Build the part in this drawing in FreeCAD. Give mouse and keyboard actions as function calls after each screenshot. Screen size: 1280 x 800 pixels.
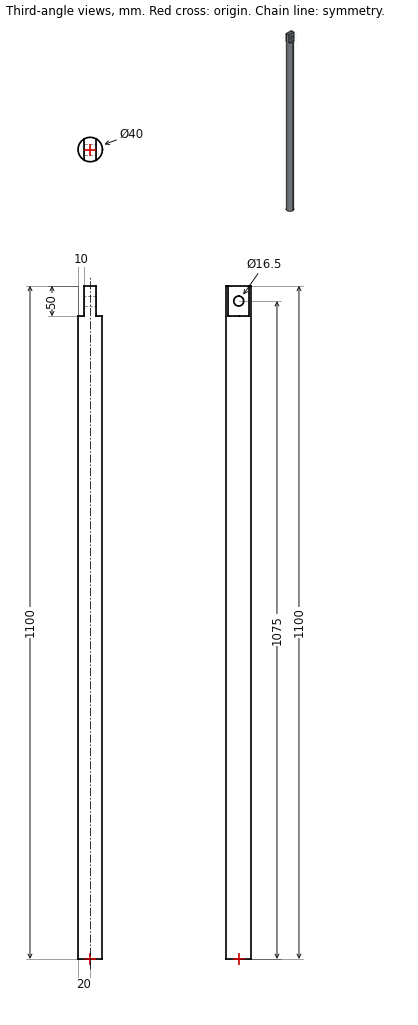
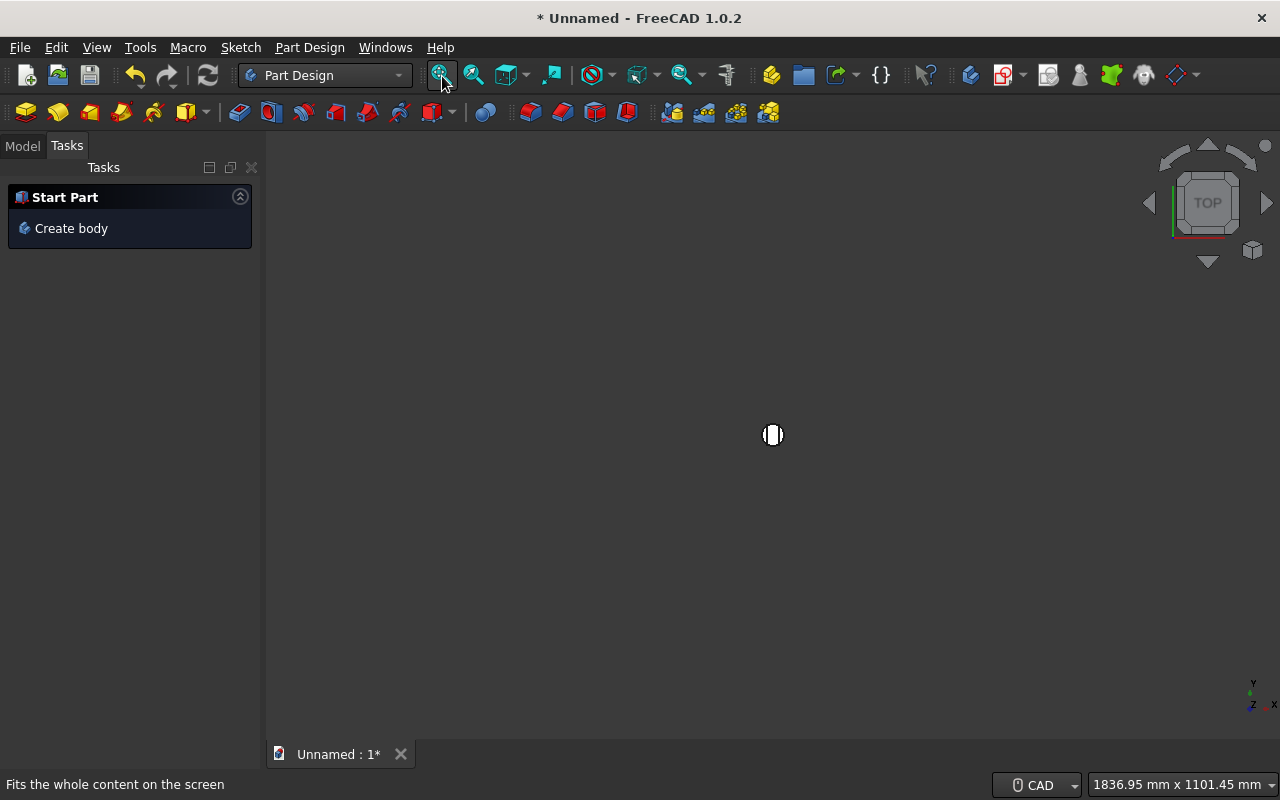
click(442, 76)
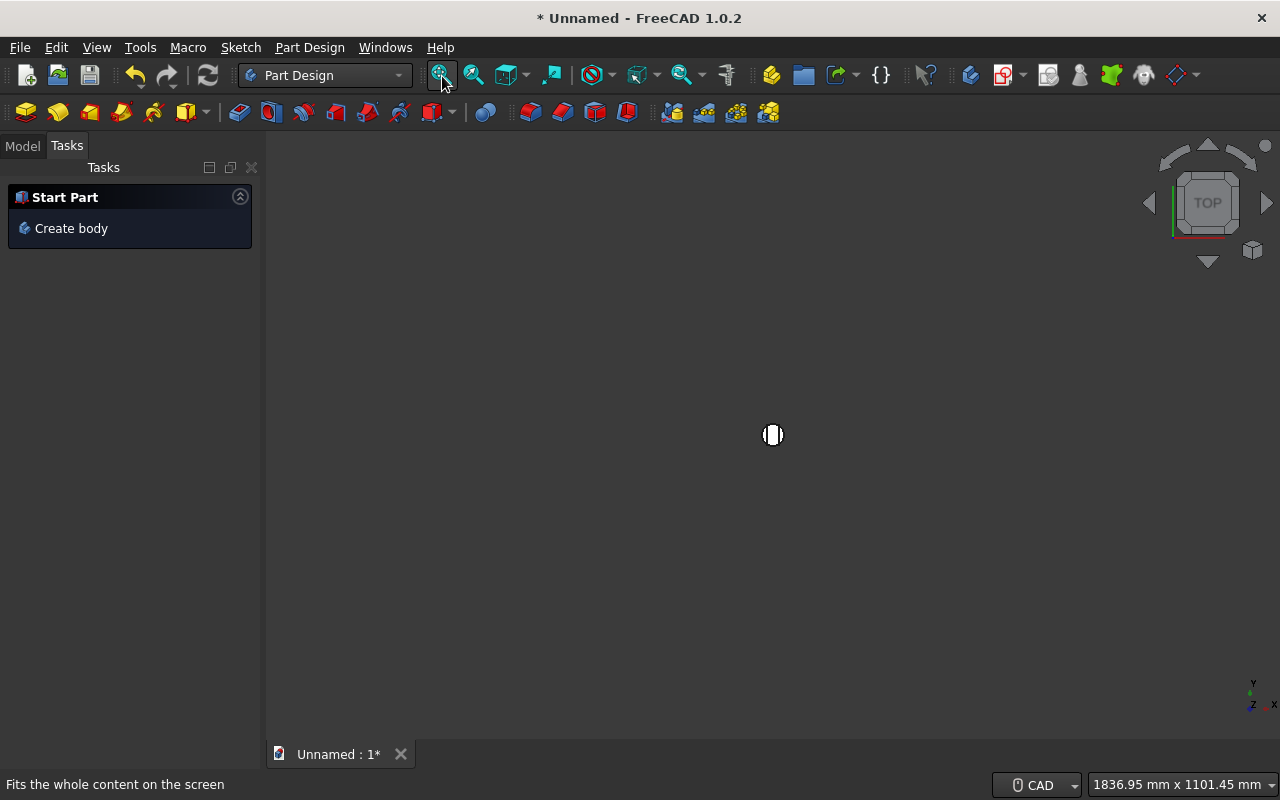
key(1)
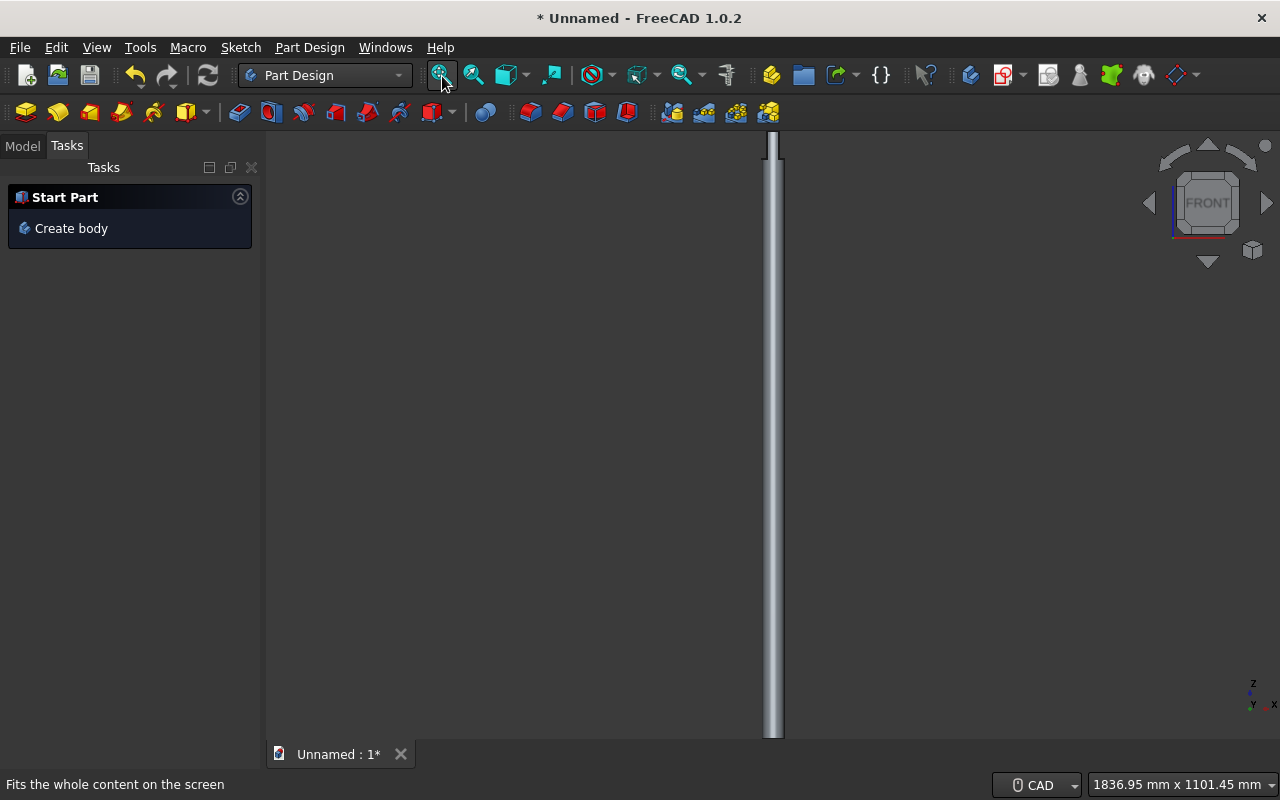
click(442, 76)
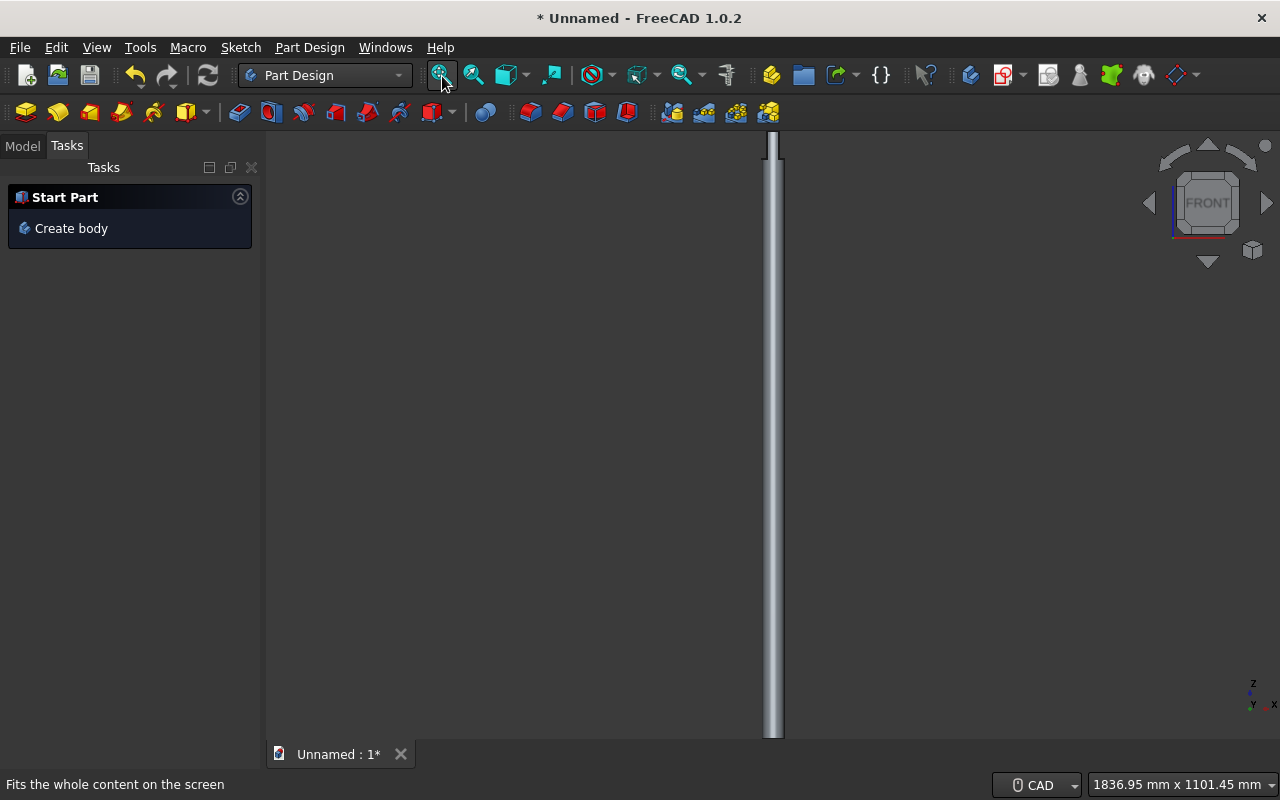
click(23, 145)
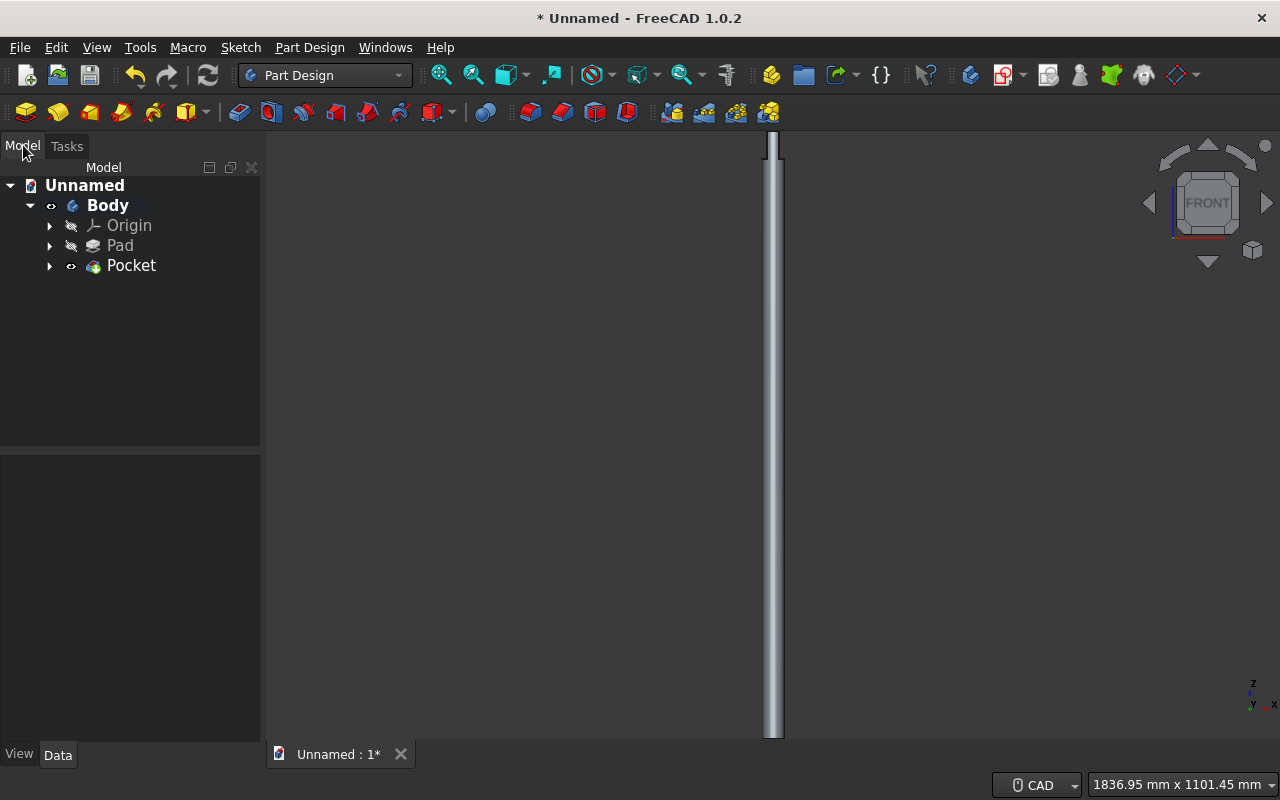
click(50, 226)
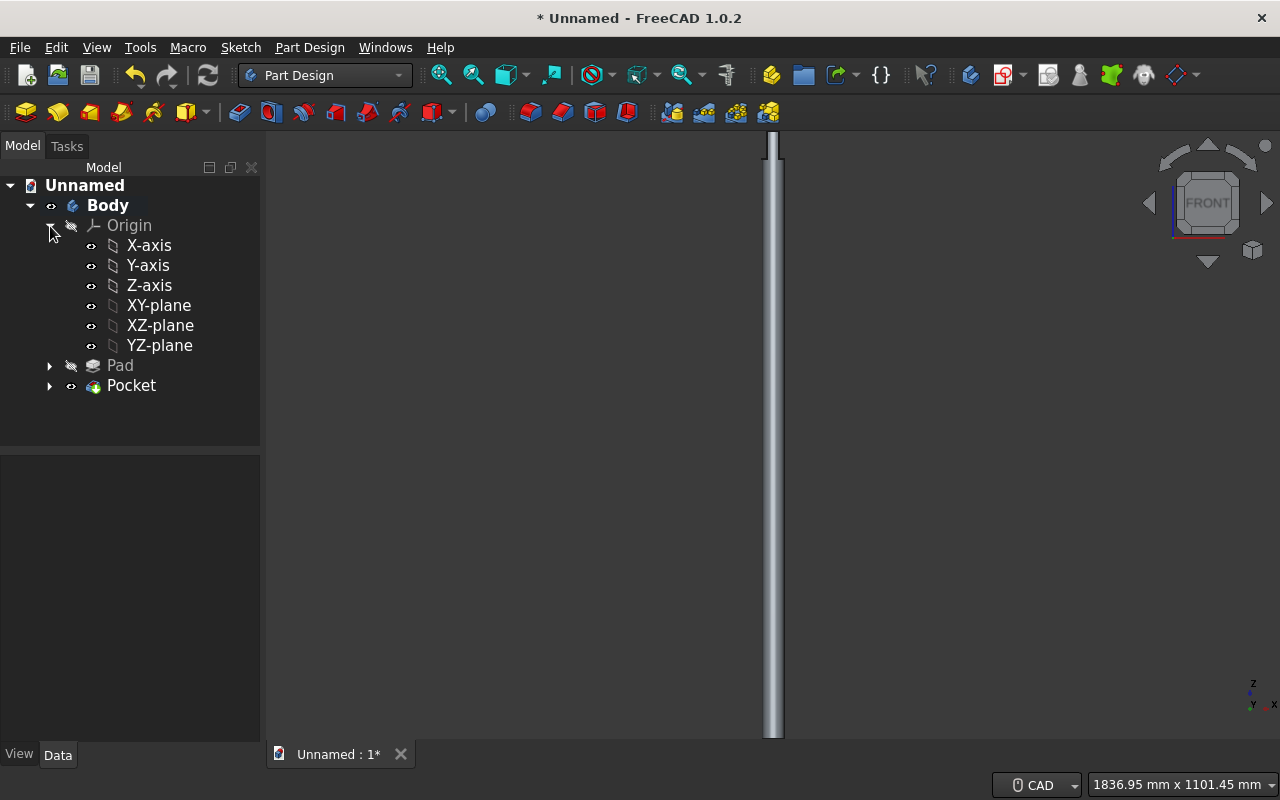
click(136, 346)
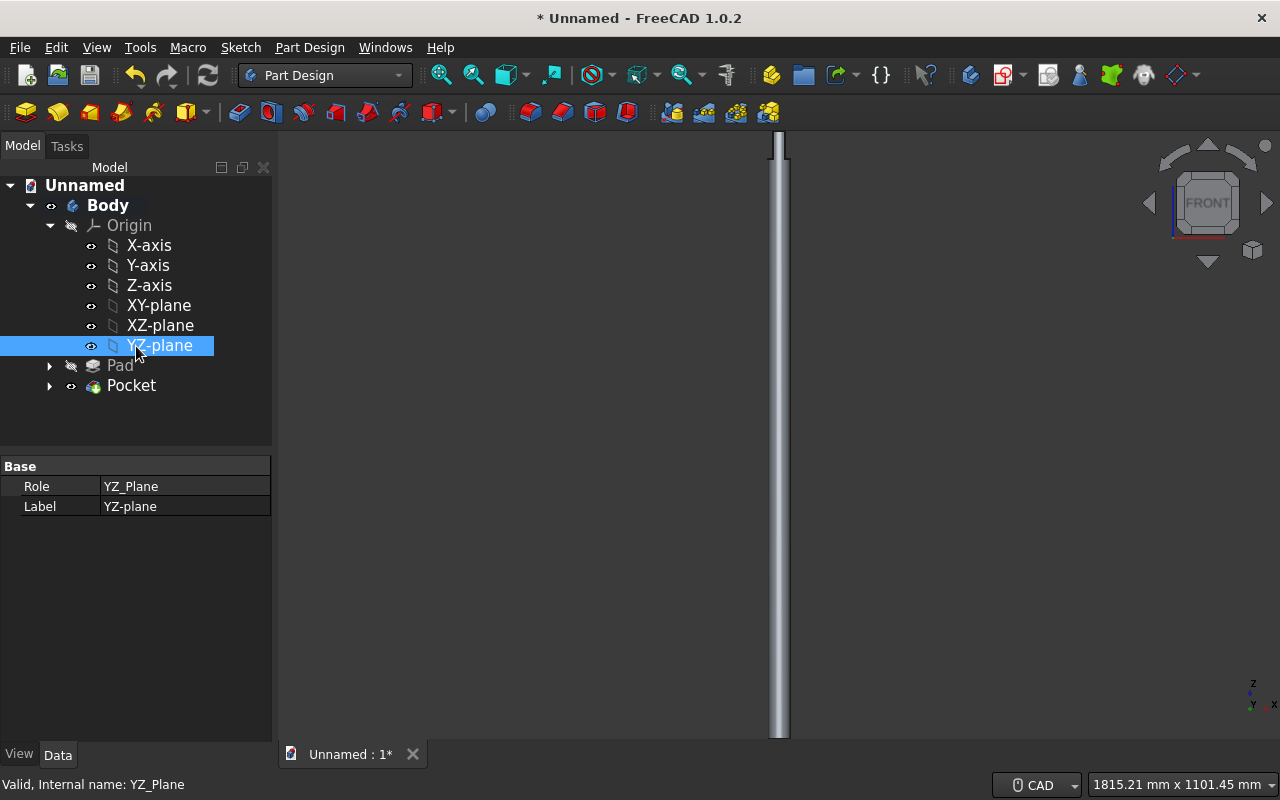
click(1176, 76)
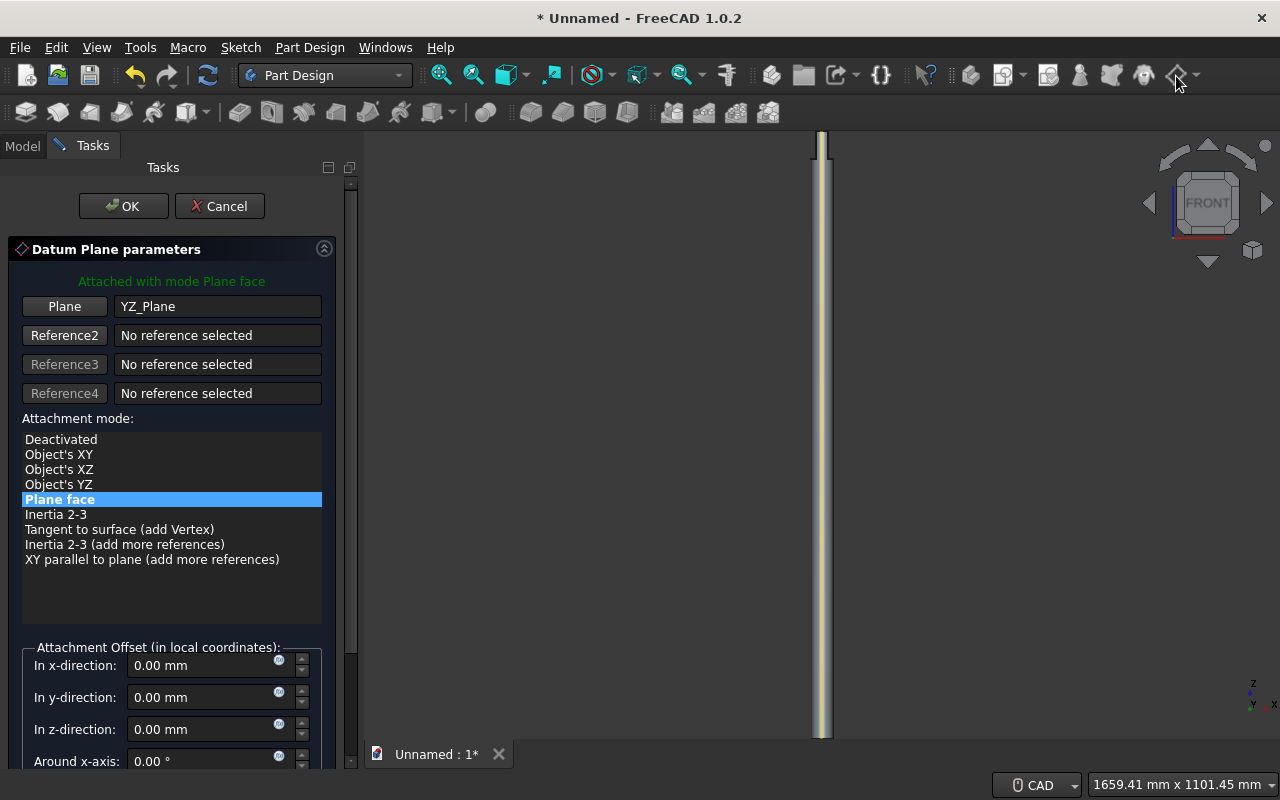
triple_click(210, 729)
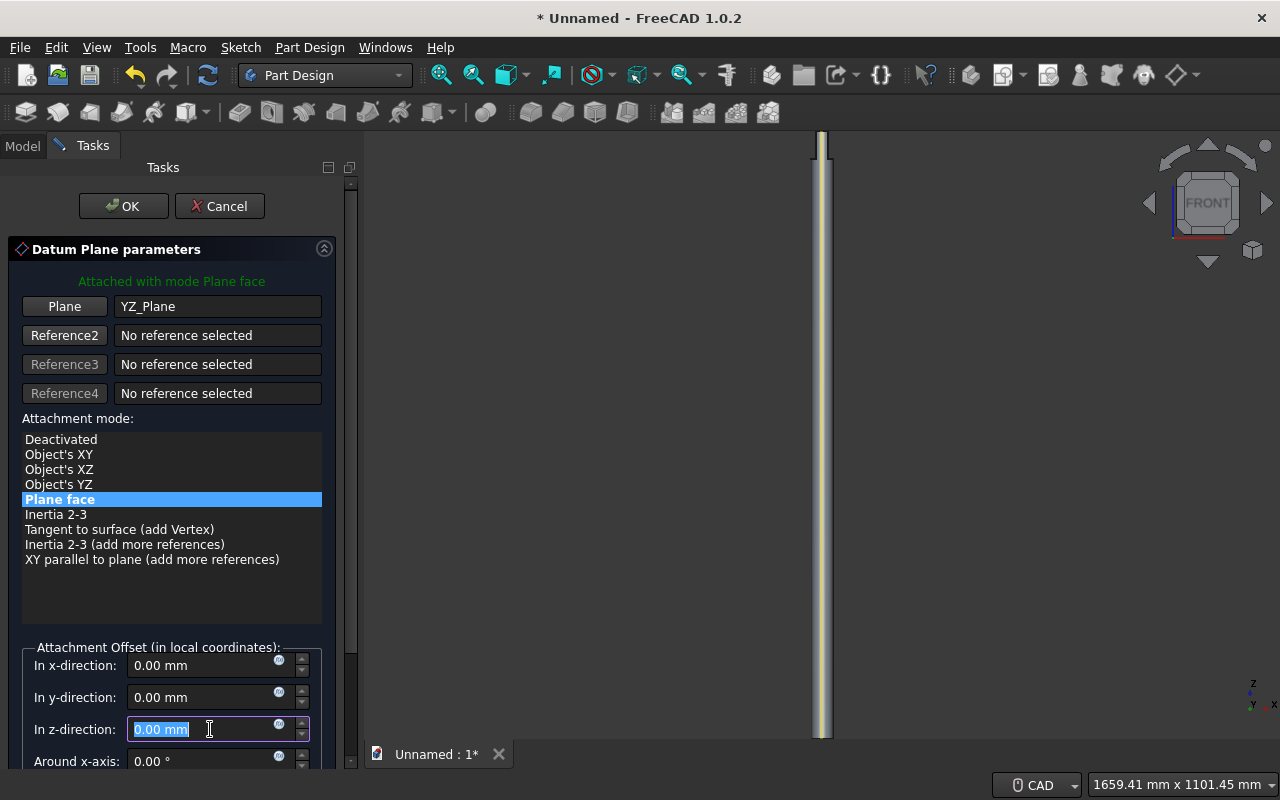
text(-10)
key(Tab)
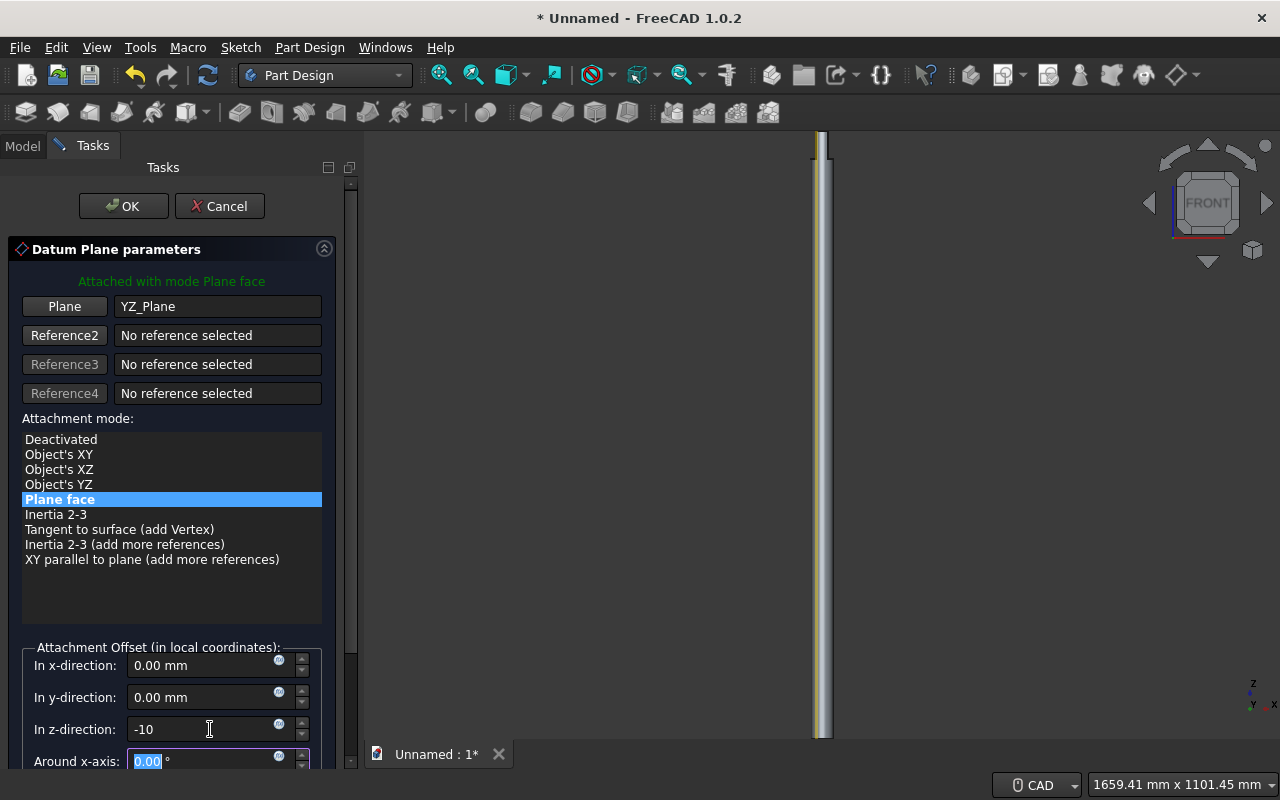
click(124, 206)